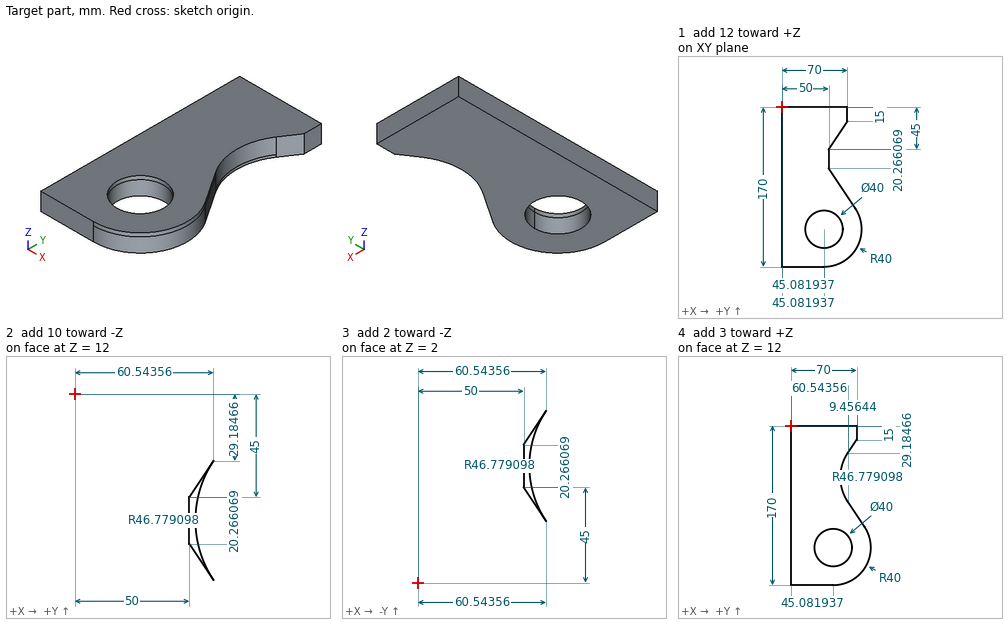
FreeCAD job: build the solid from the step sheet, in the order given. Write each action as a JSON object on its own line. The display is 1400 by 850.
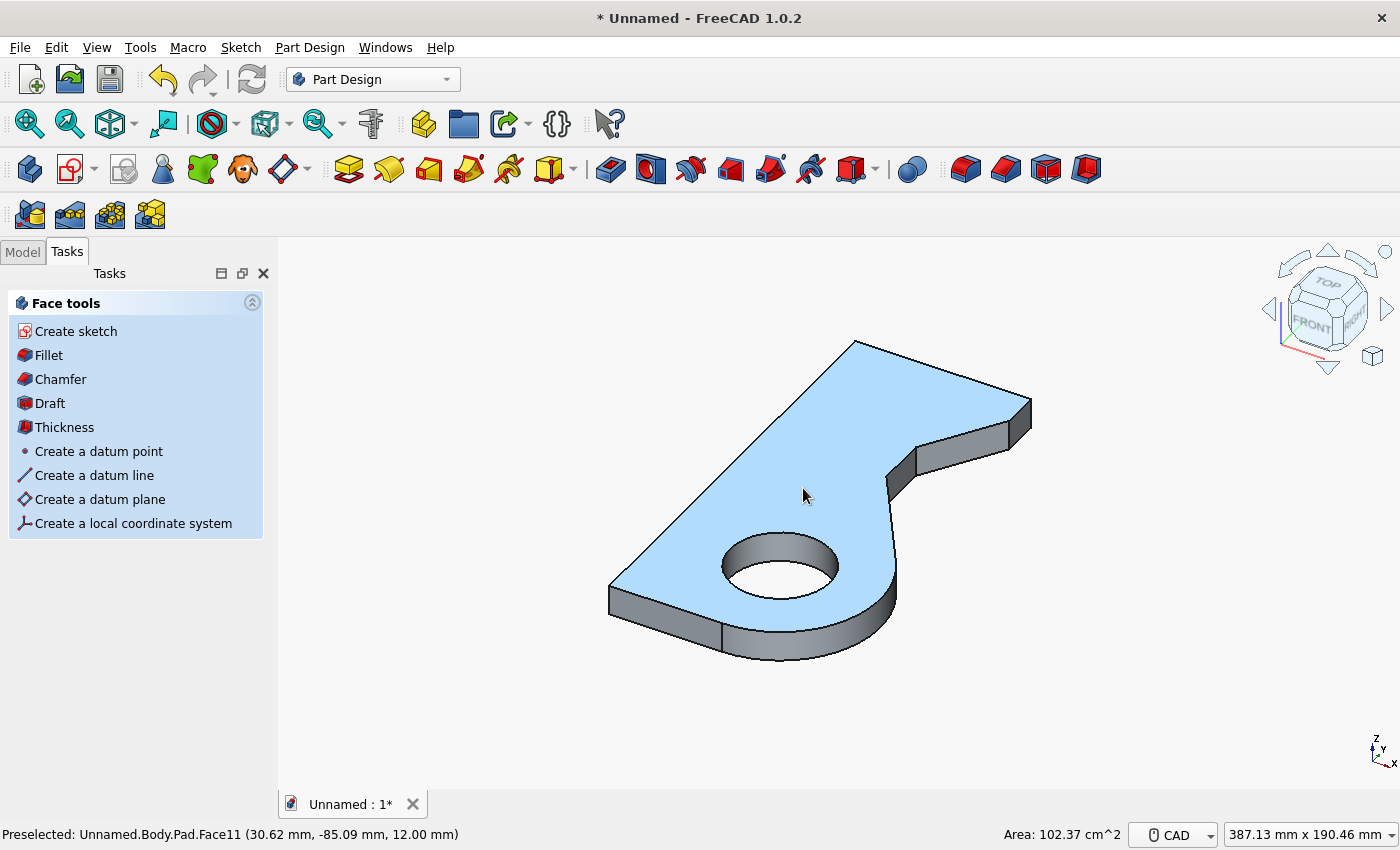
{"action": "left_click", "coordinate": [70, 170]}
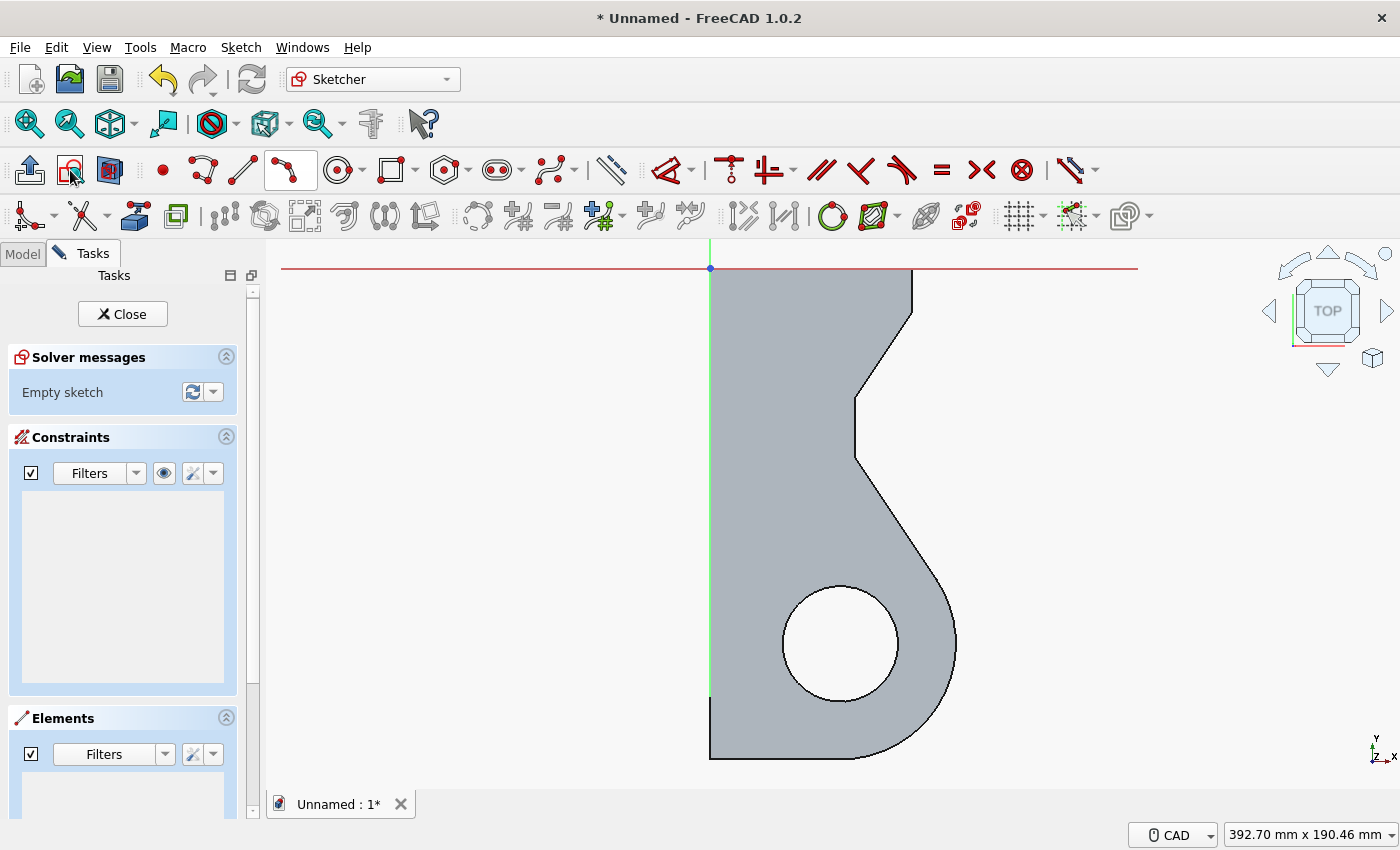
{"action": "scroll", "coordinate": [615, 761], "scroll_direction": "down", "scroll_amount": 1}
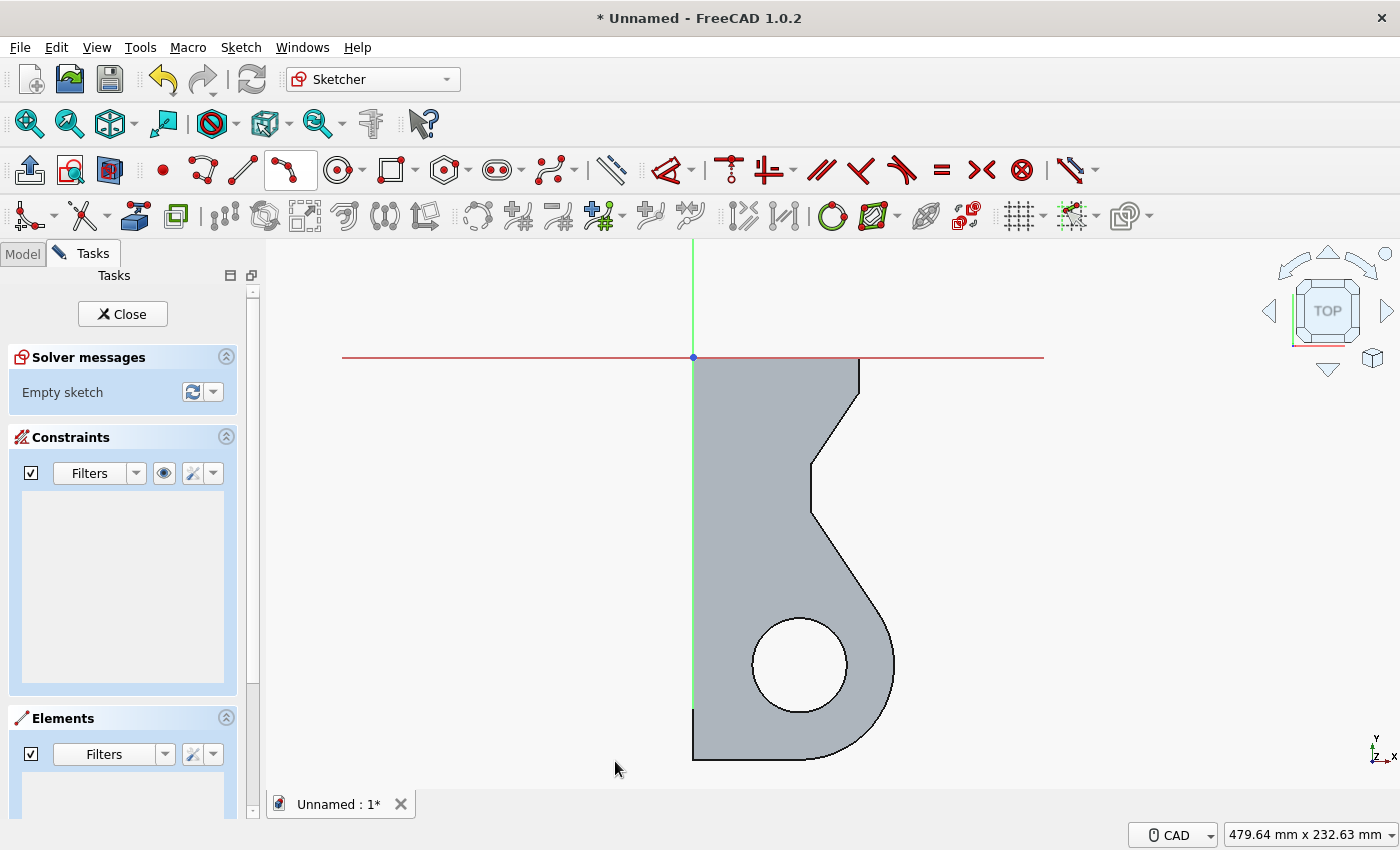
{"action": "scroll", "coordinate": [765, 381], "scroll_direction": "up", "scroll_amount": 3}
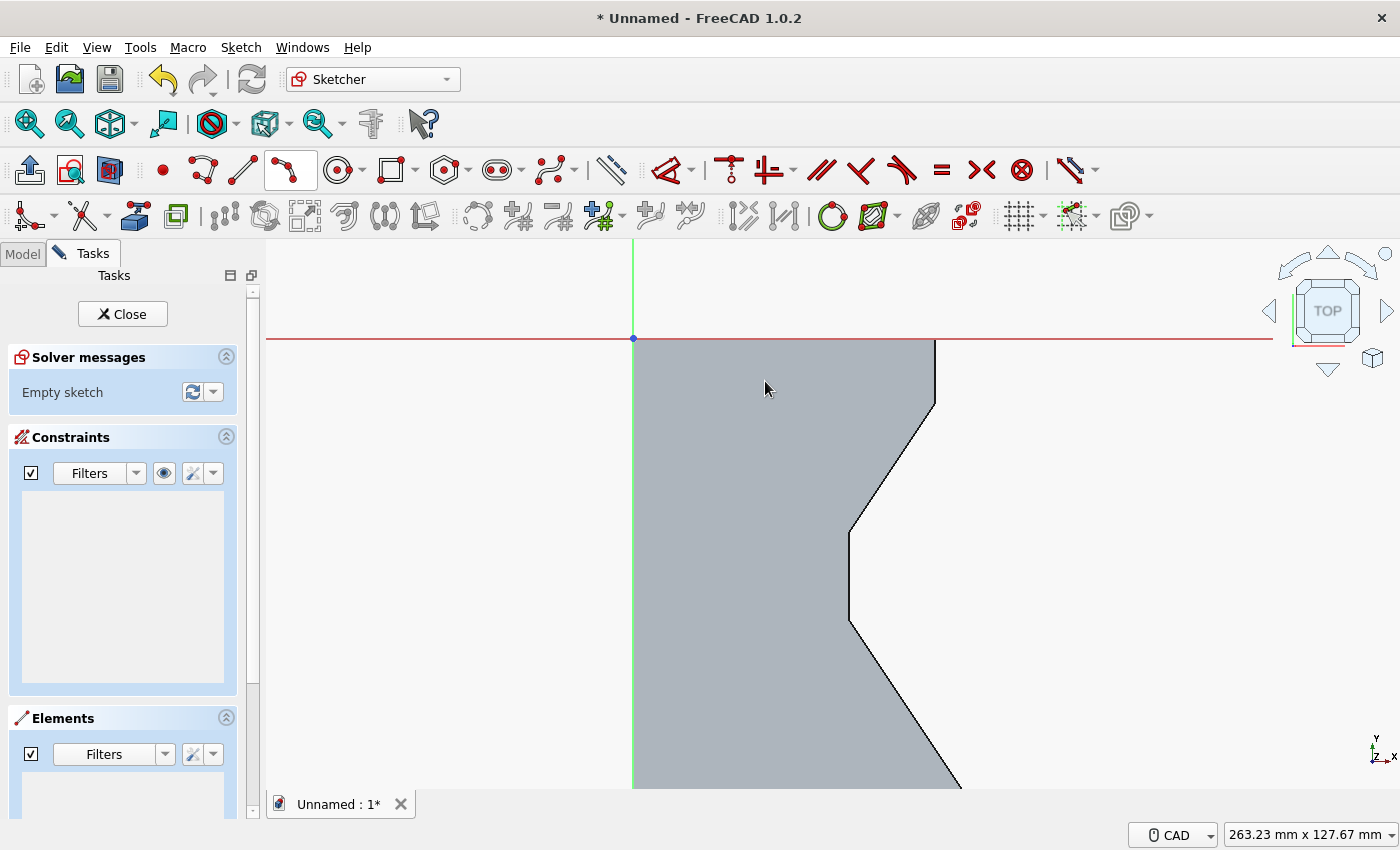
{"action": "left_click", "coordinate": [204, 170]}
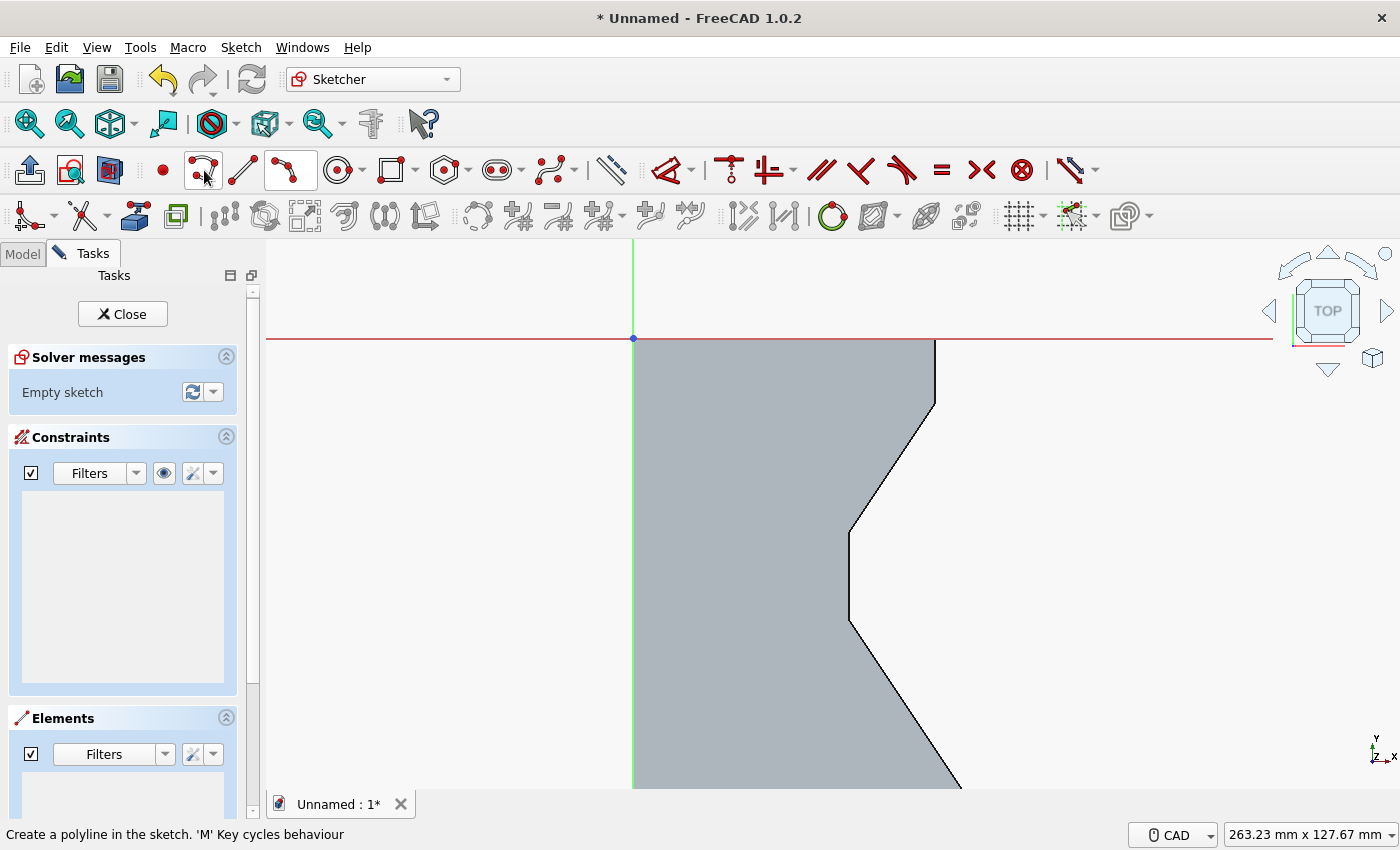
{"action": "left_click", "coordinate": [894, 465]}
{"action": "left_click", "coordinate": [849, 533]}
{"action": "left_click", "coordinate": [849, 620]}
{"action": "left_click", "coordinate": [894, 688]}
{"action": "right_click", "coordinate": [894, 688]}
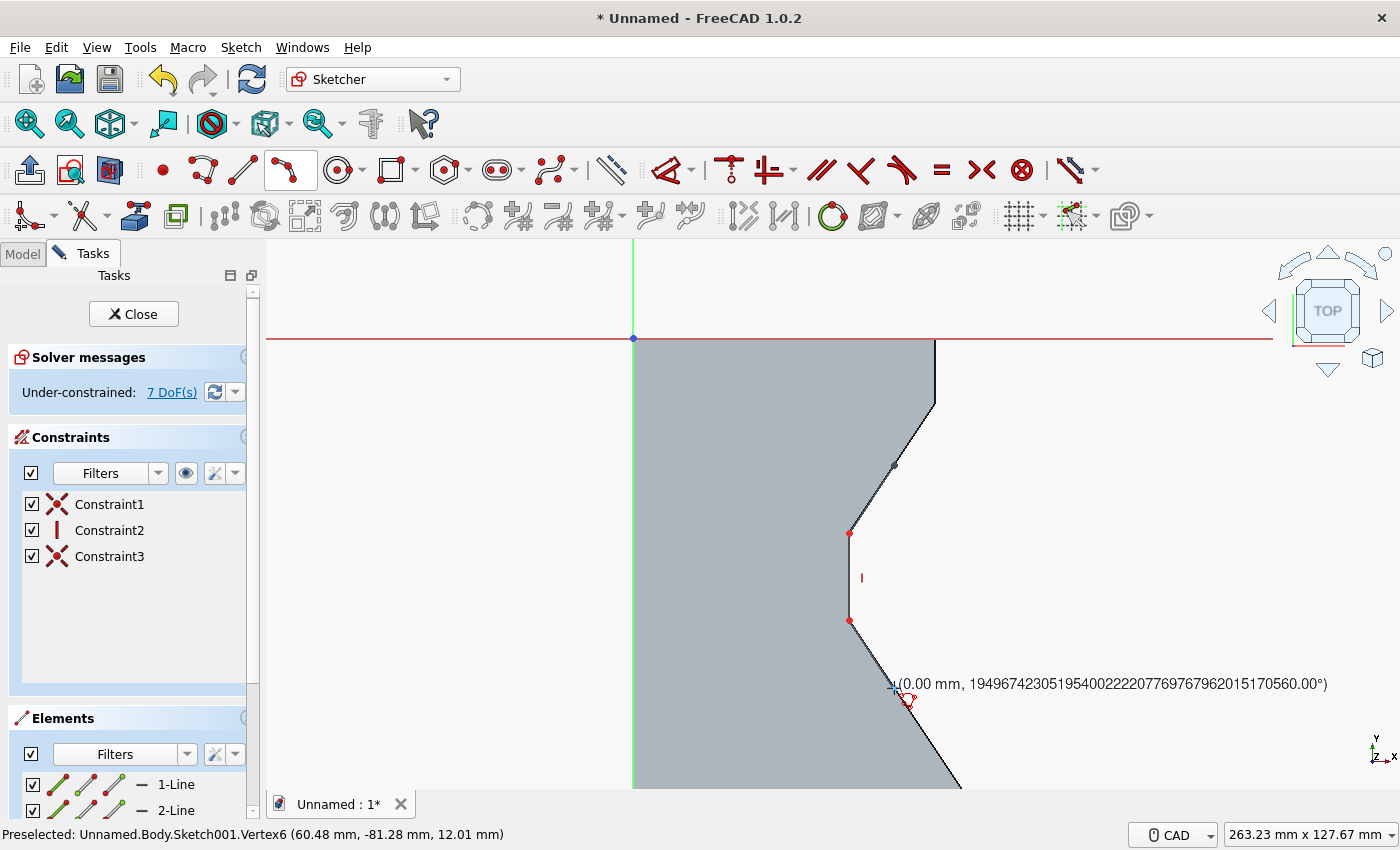
{"action": "left_click", "coordinate": [284, 170]}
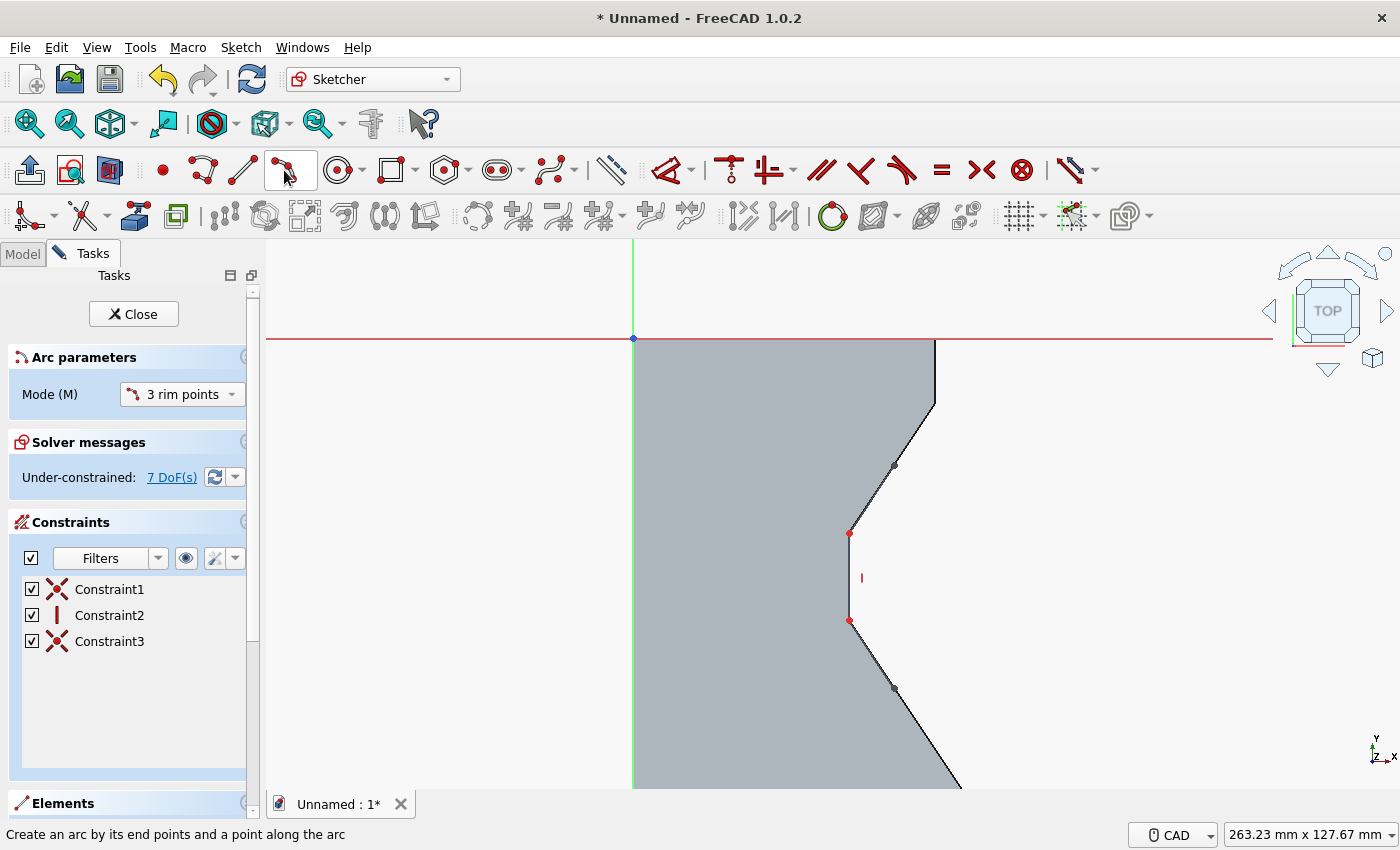
{"action": "left_click", "coordinate": [894, 689]}
{"action": "left_click", "coordinate": [894, 466]}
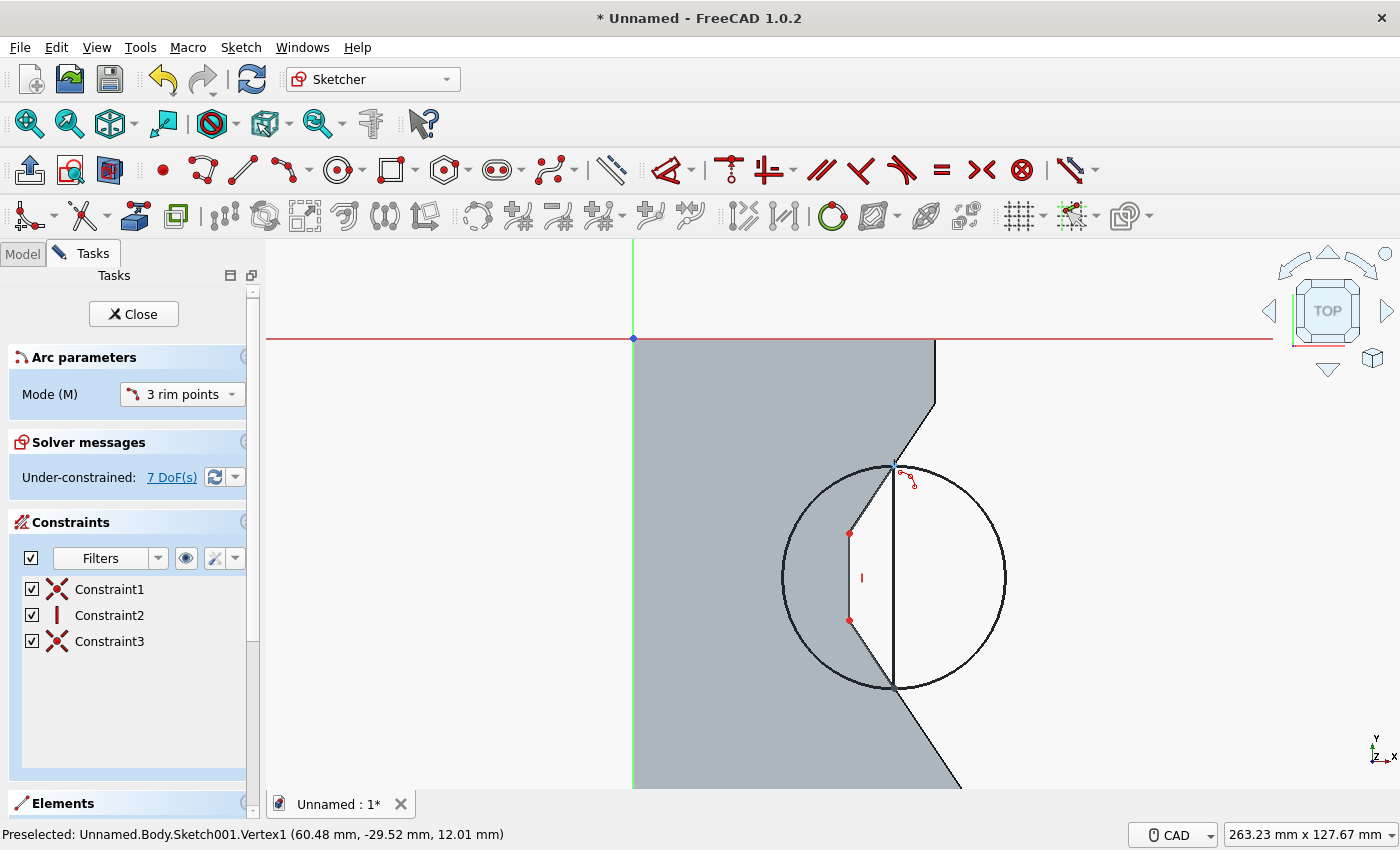
{"action": "scroll", "coordinate": [862, 600], "scroll_direction": "up", "scroll_amount": 2}